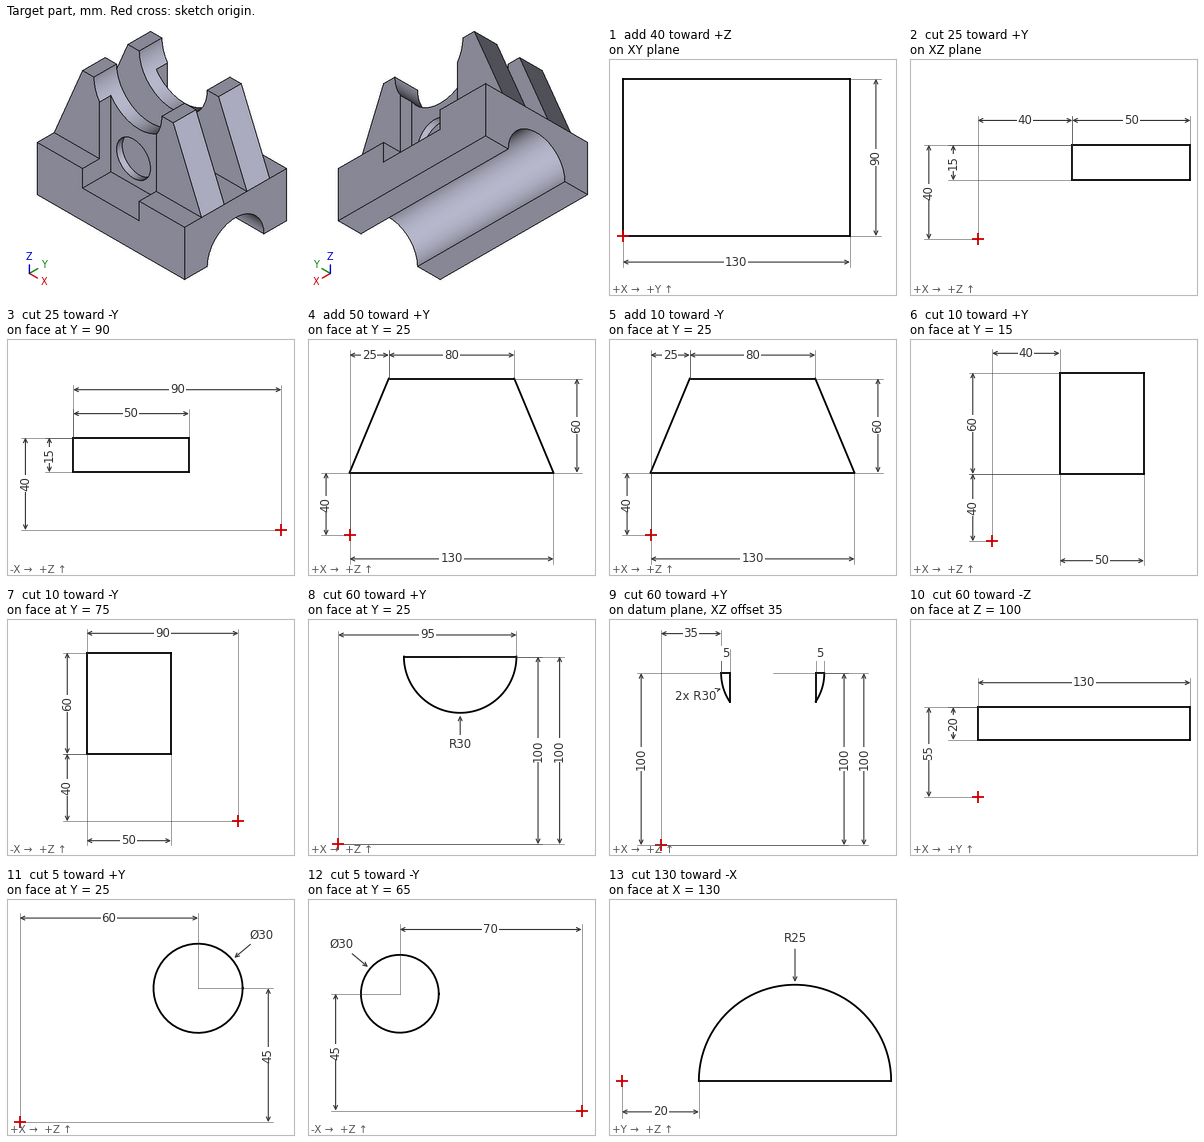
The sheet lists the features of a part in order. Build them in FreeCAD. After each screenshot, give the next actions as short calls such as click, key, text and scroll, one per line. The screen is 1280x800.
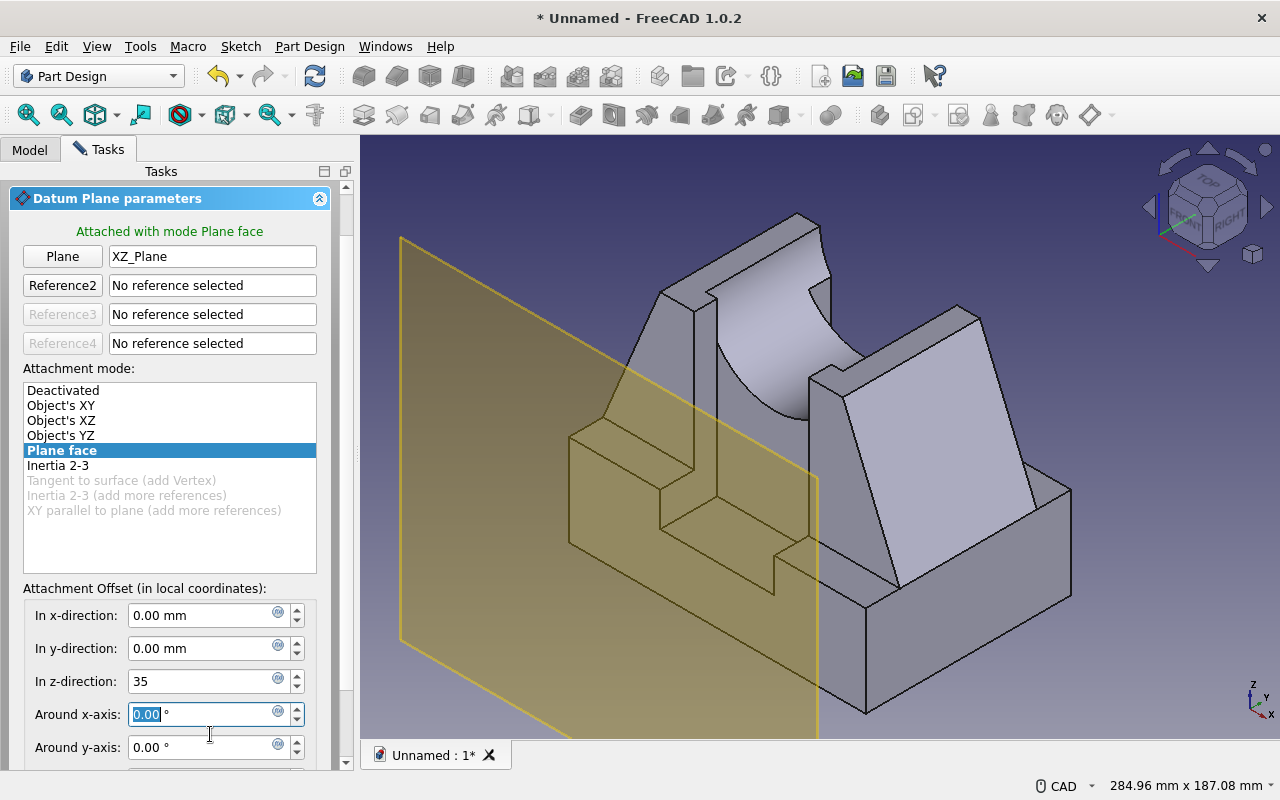
scroll(346, 476, up, 2)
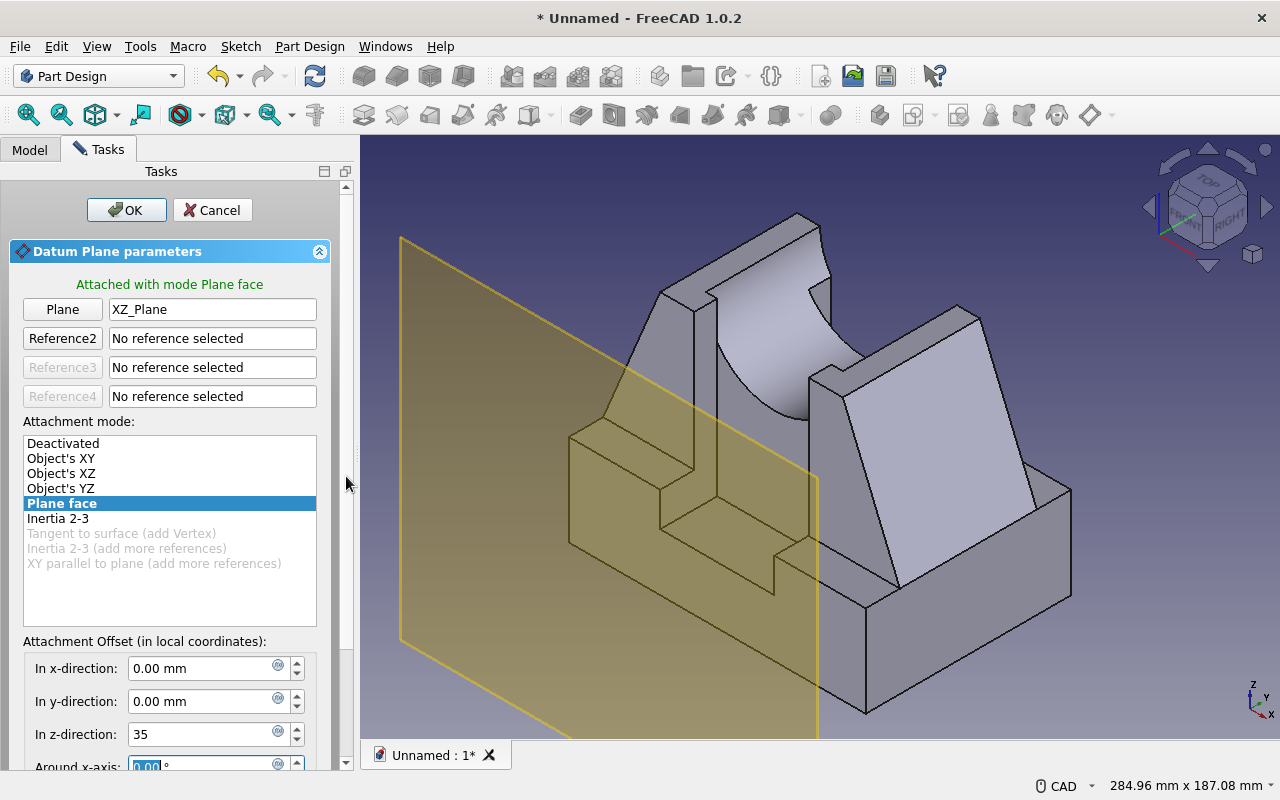
click(127, 210)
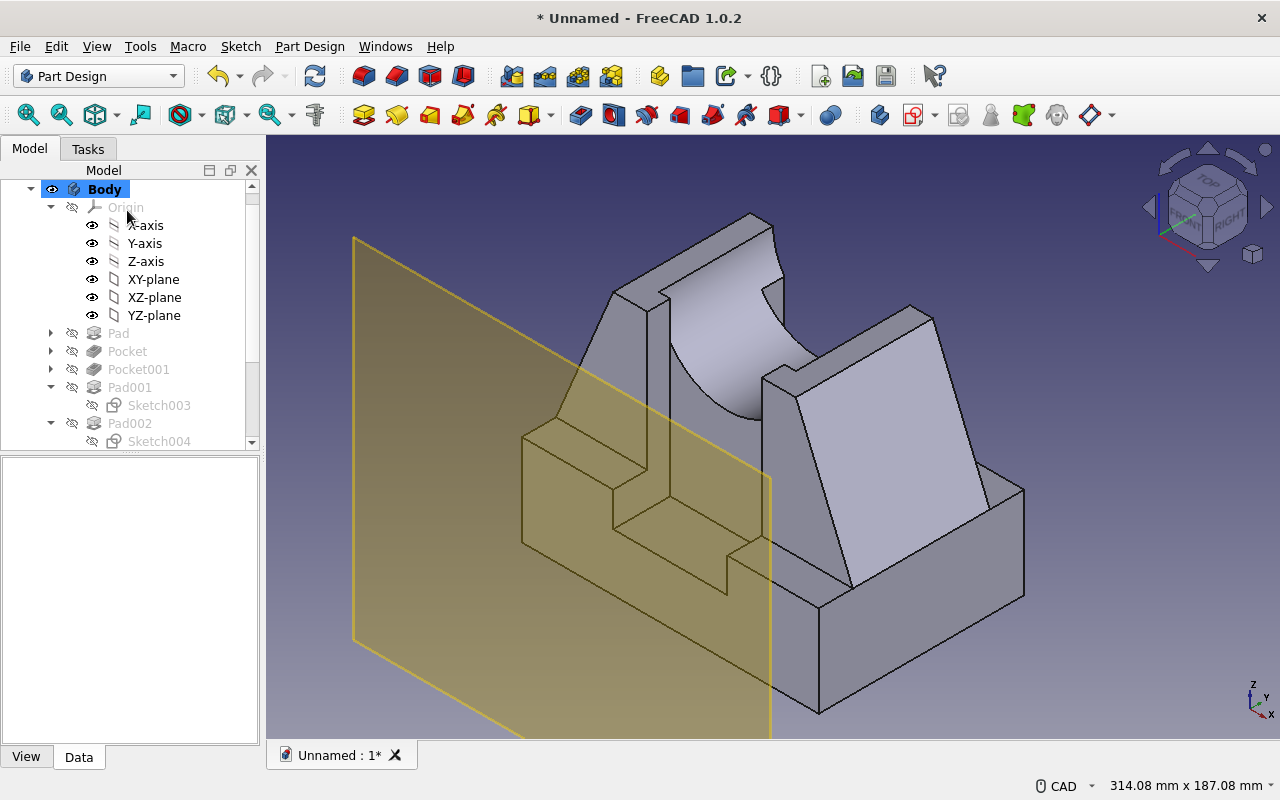
scroll(121, 311, down, 3)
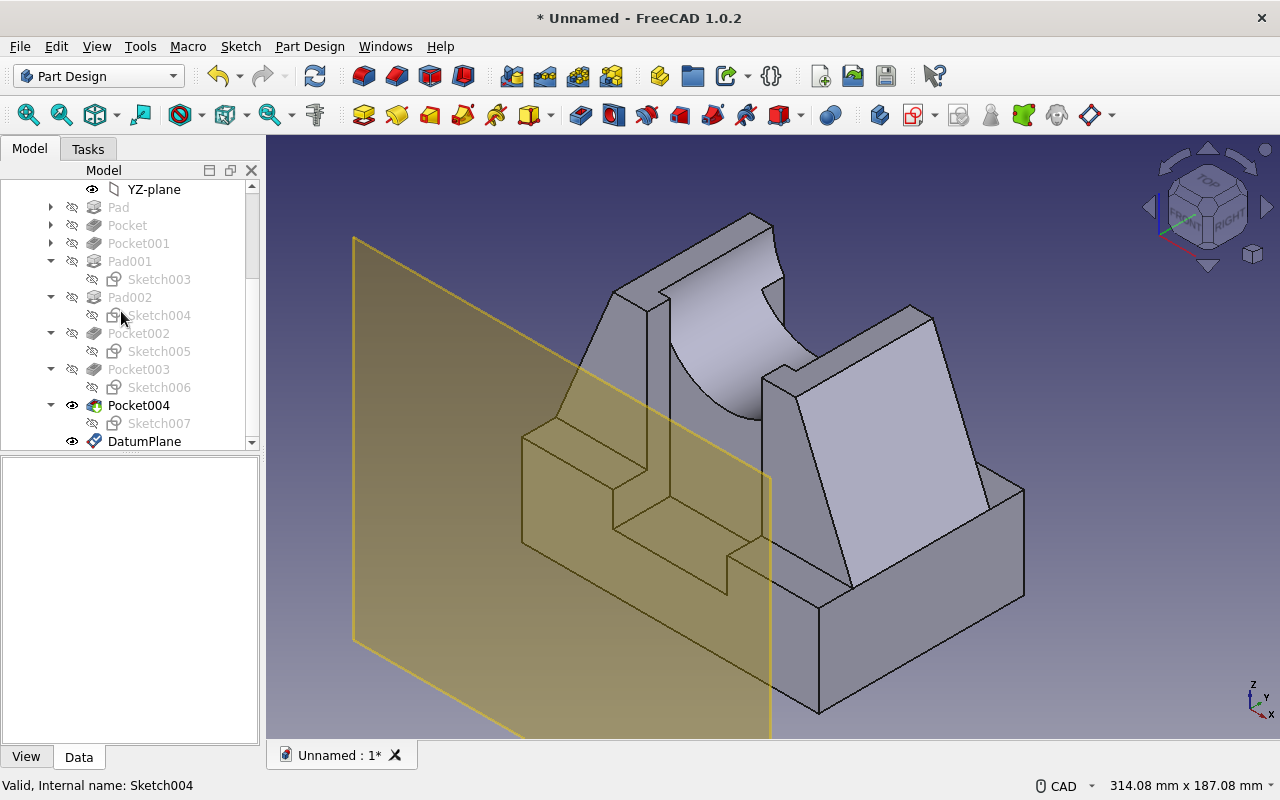
click(117, 441)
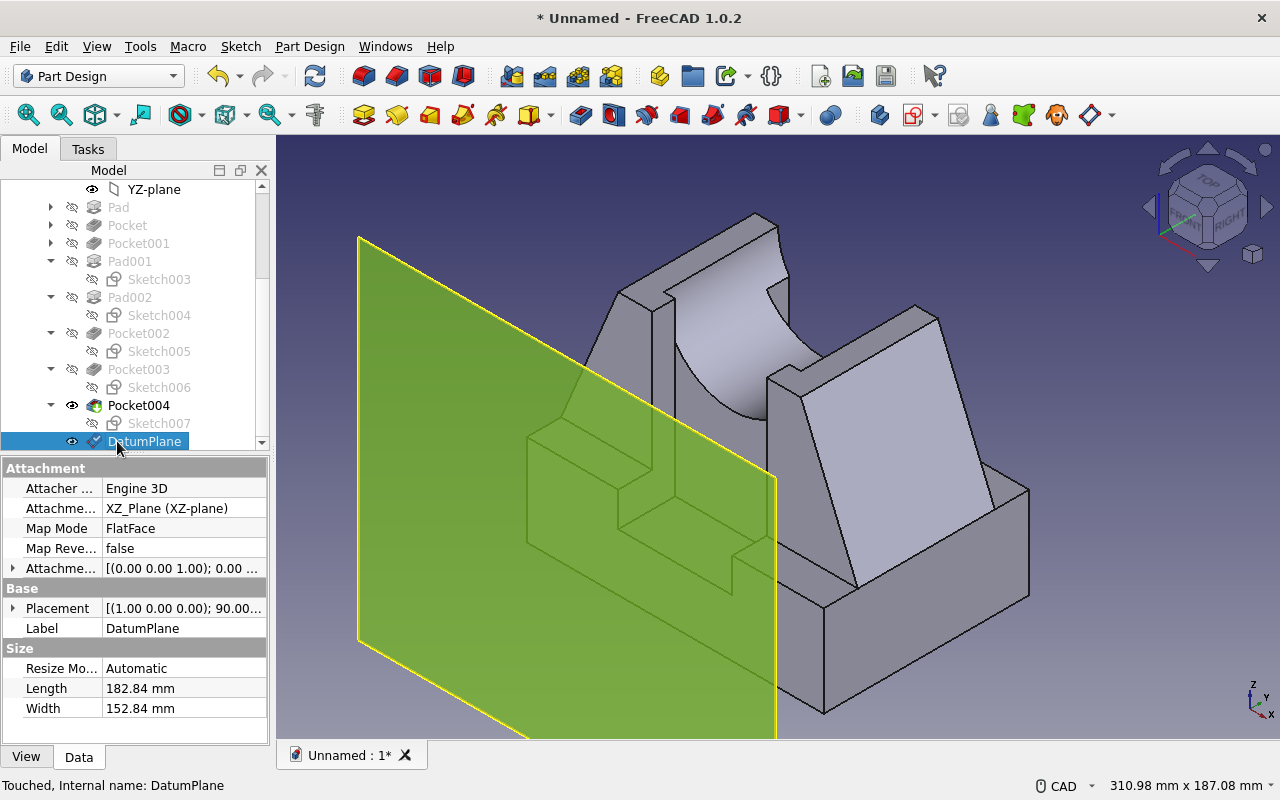
click(912, 116)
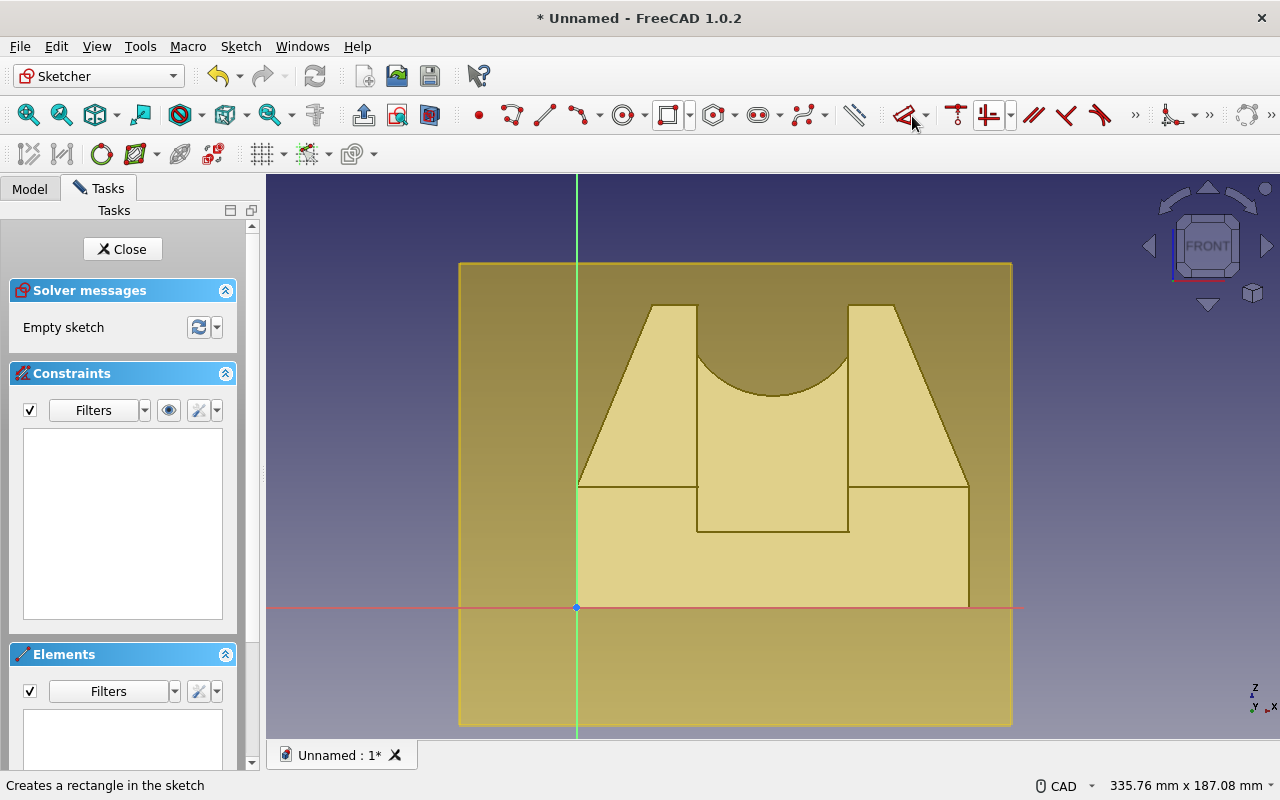
key(g)
key(m)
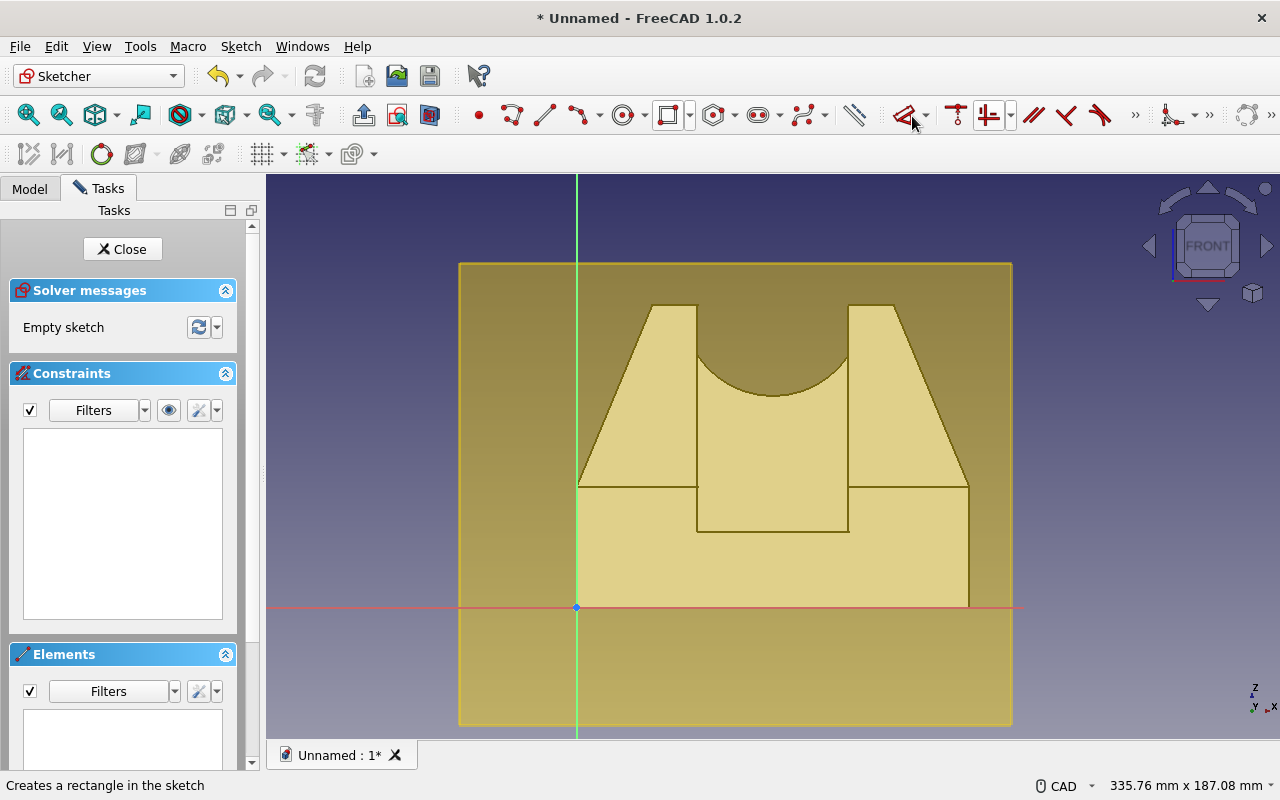
click(682, 305)
click(697, 305)
click(697, 356)
right_click(697, 356)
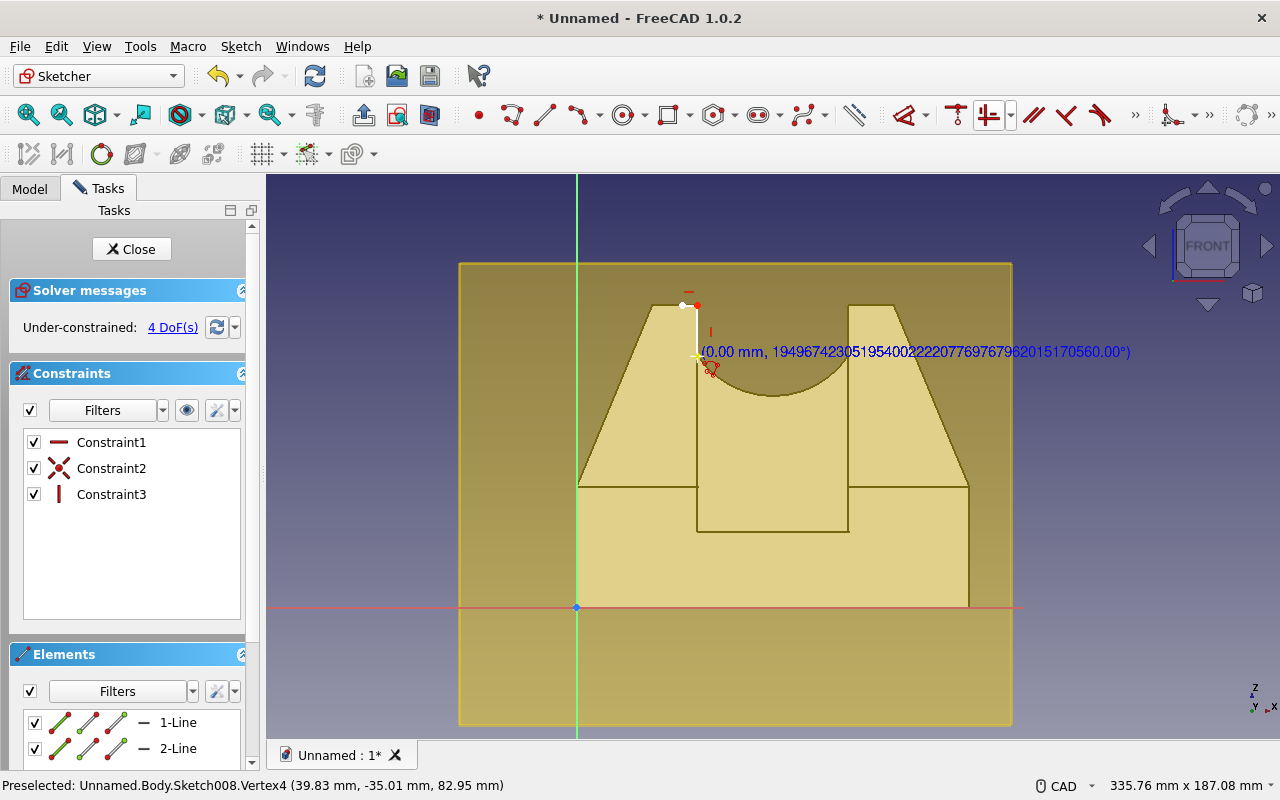
key(g)
key(3)
key(a)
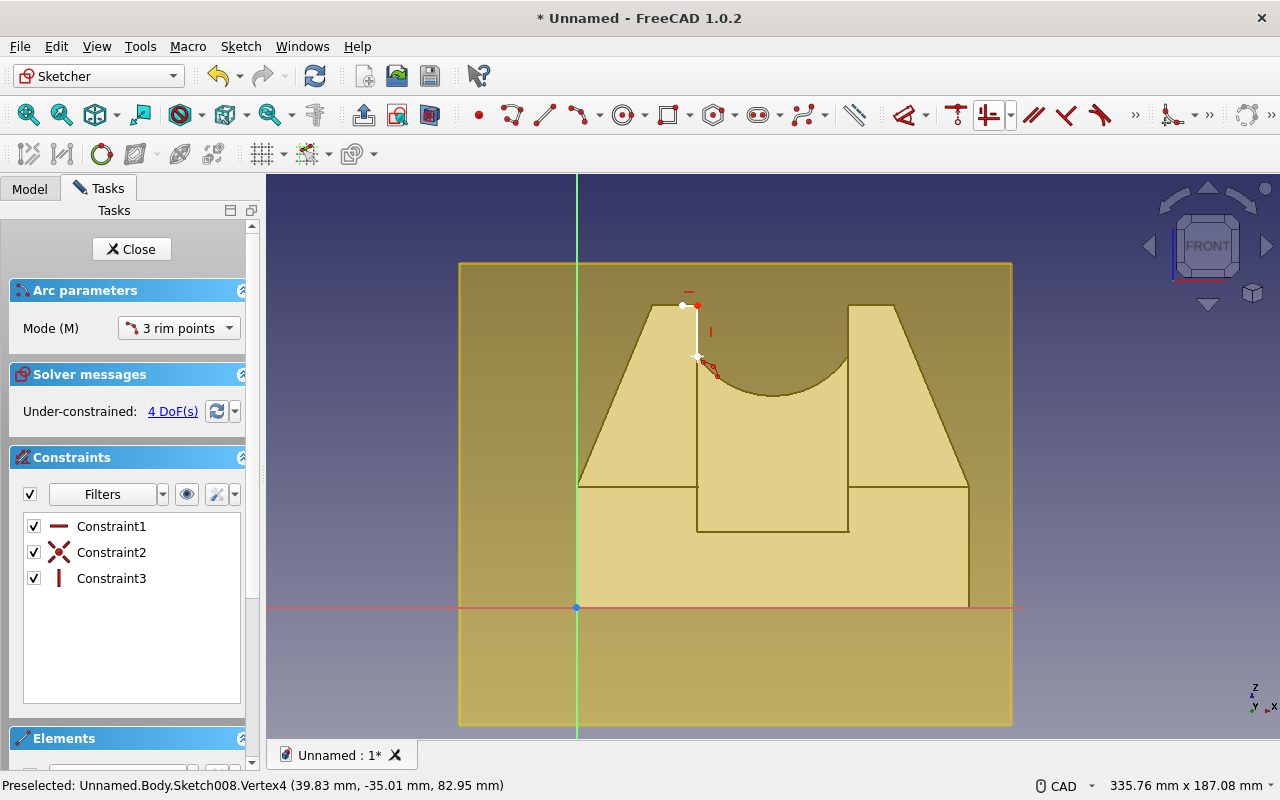
click(697, 357)